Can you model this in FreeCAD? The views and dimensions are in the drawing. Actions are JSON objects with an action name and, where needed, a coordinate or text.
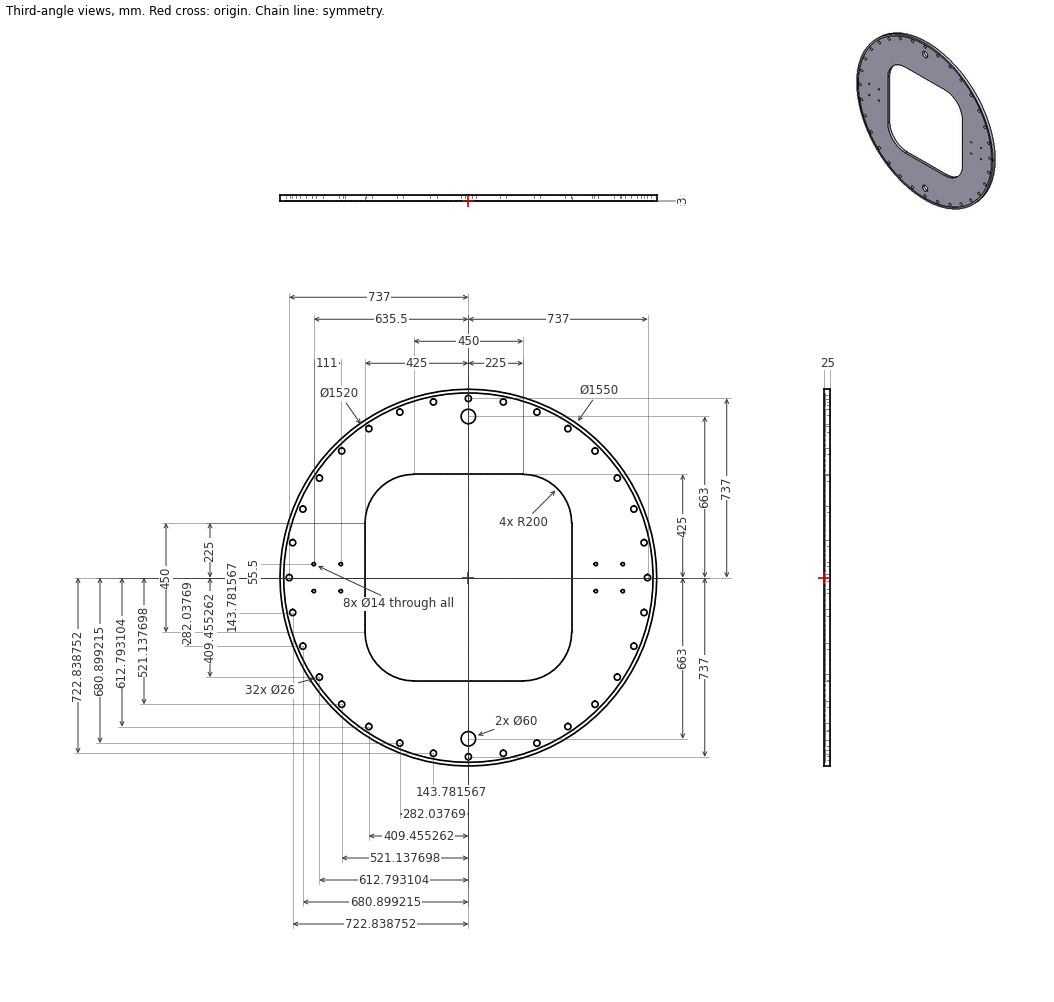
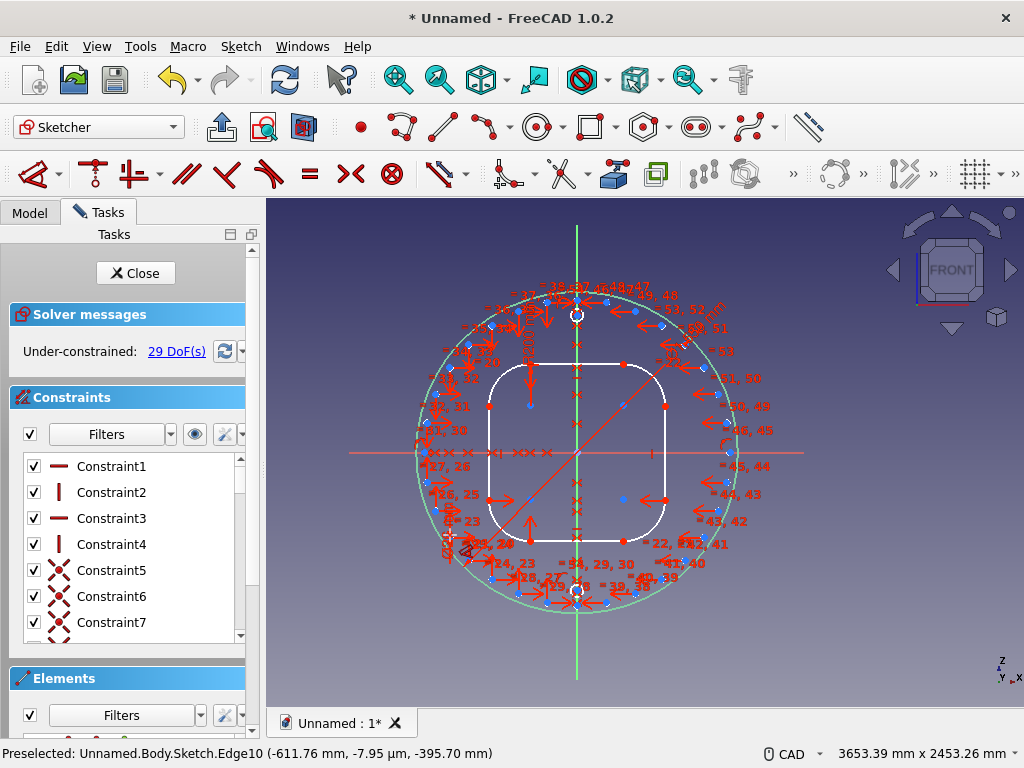
{"action": "scroll", "coordinate": [581, 586], "scroll_direction": "up", "scroll_amount": 6}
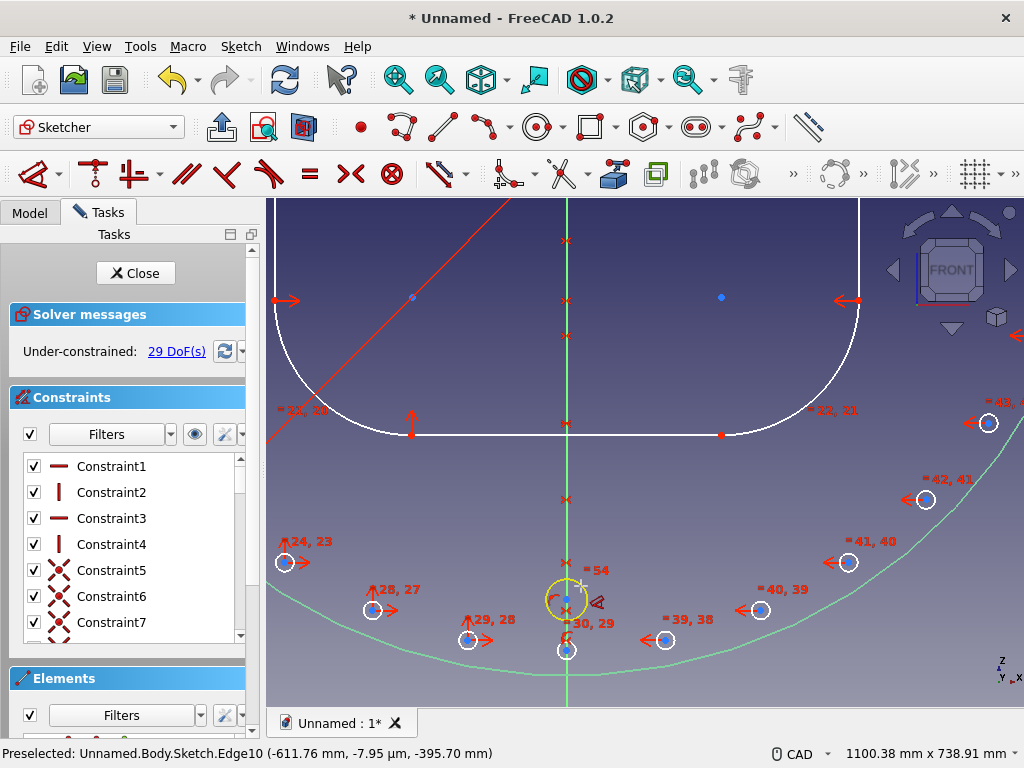
{"action": "left_click", "coordinate": [581, 585]}
{"action": "left_click", "coordinate": [603, 562]}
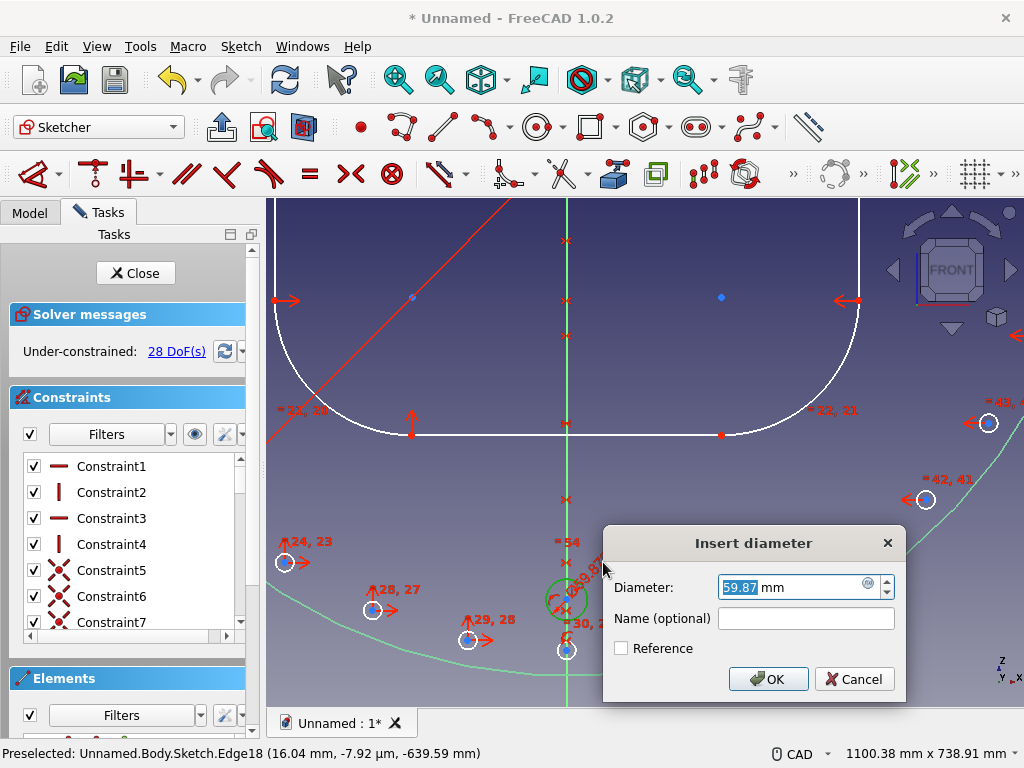
{"action": "type", "text": "60"}
{"action": "key", "text": "Return"}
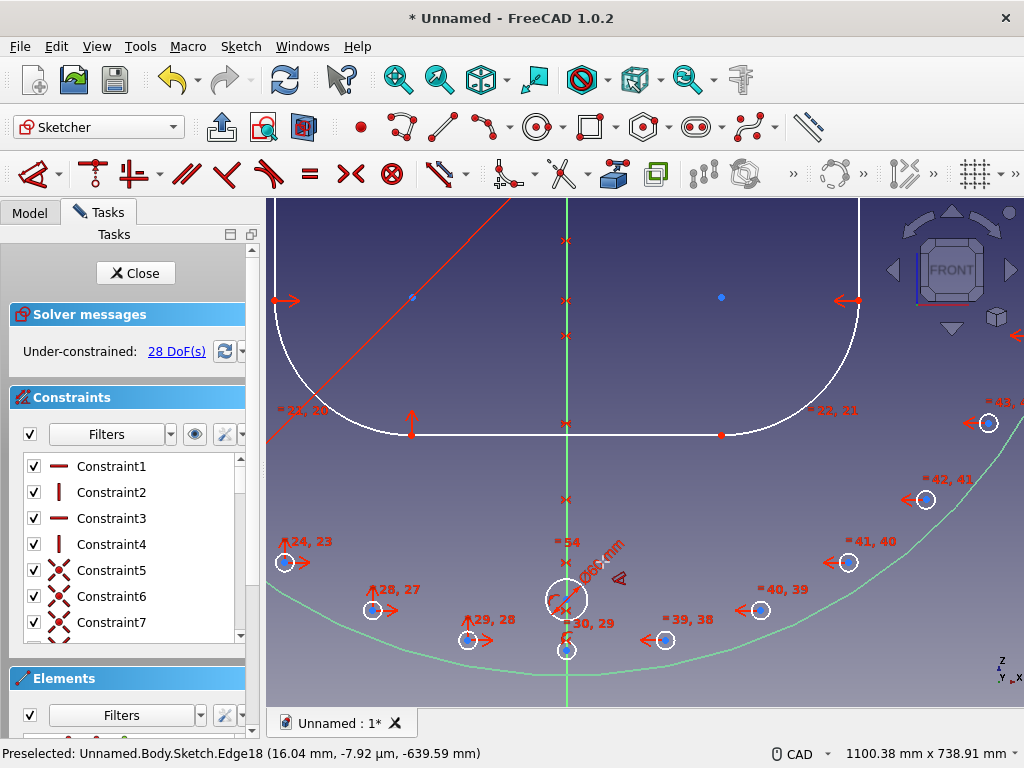
{"action": "scroll", "coordinate": [581, 586], "scroll_direction": "down", "scroll_amount": 6}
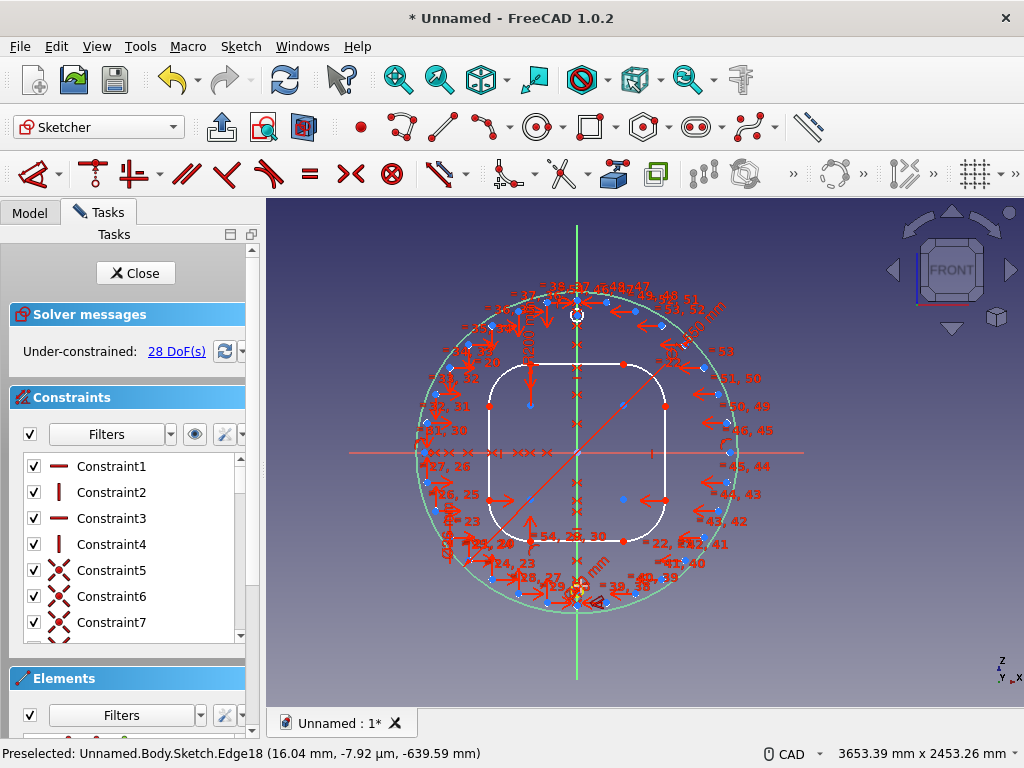
{"action": "left_click", "coordinate": [596, 364]}
{"action": "left_click", "coordinate": [610, 330]}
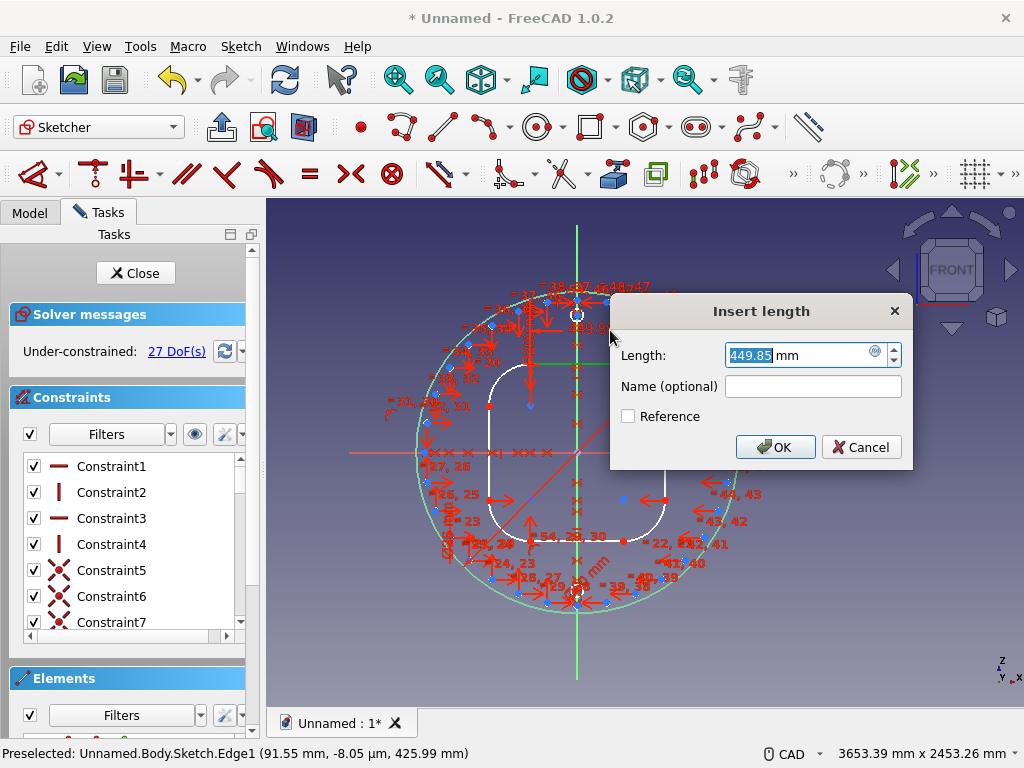
{"action": "type", "text": "450"}
{"action": "key", "text": "Return"}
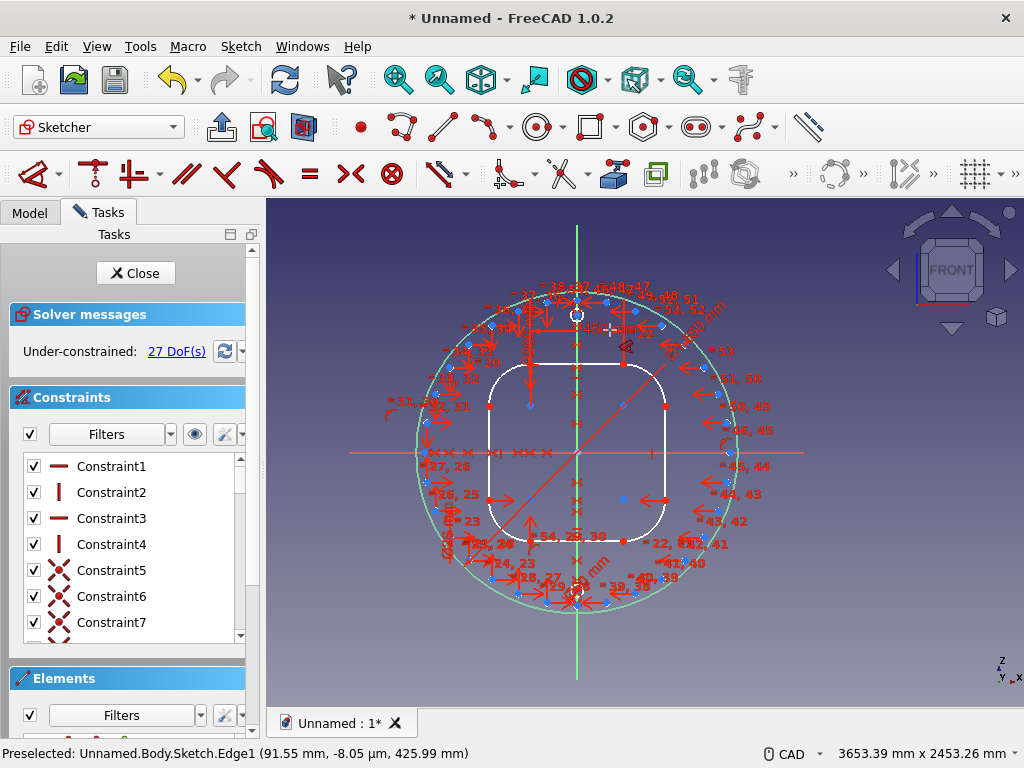
{"action": "left_click", "coordinate": [489, 435]}
{"action": "left_click", "coordinate": [455, 432]}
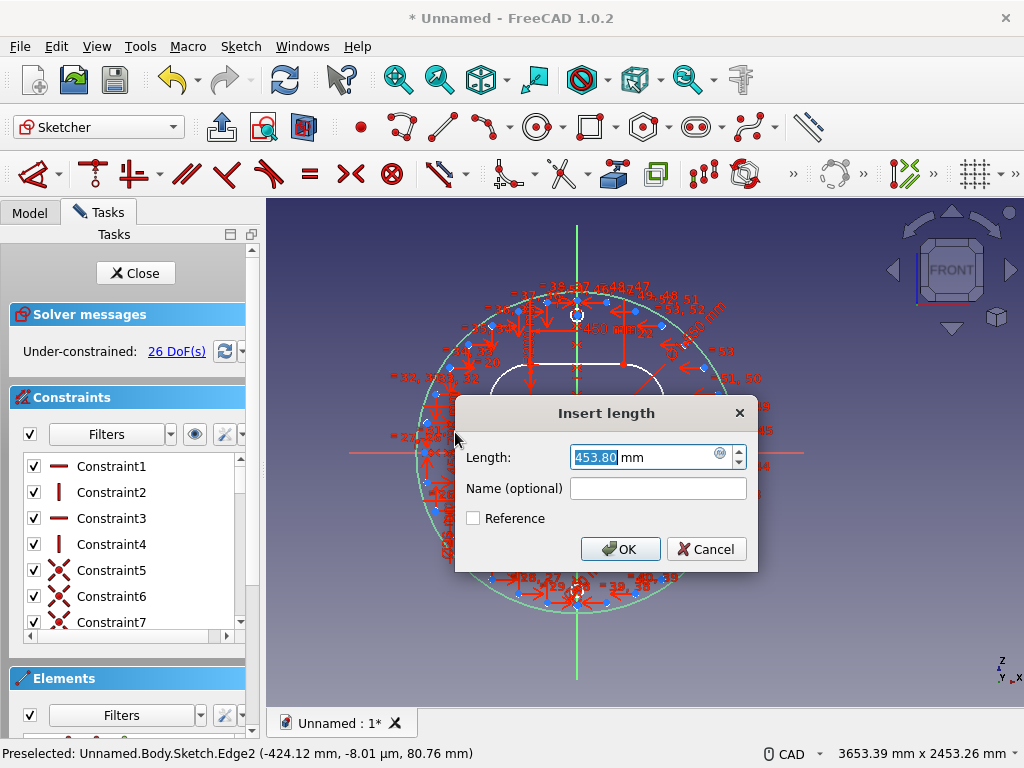
{"action": "type", "text": "450"}
{"action": "key", "text": "Return"}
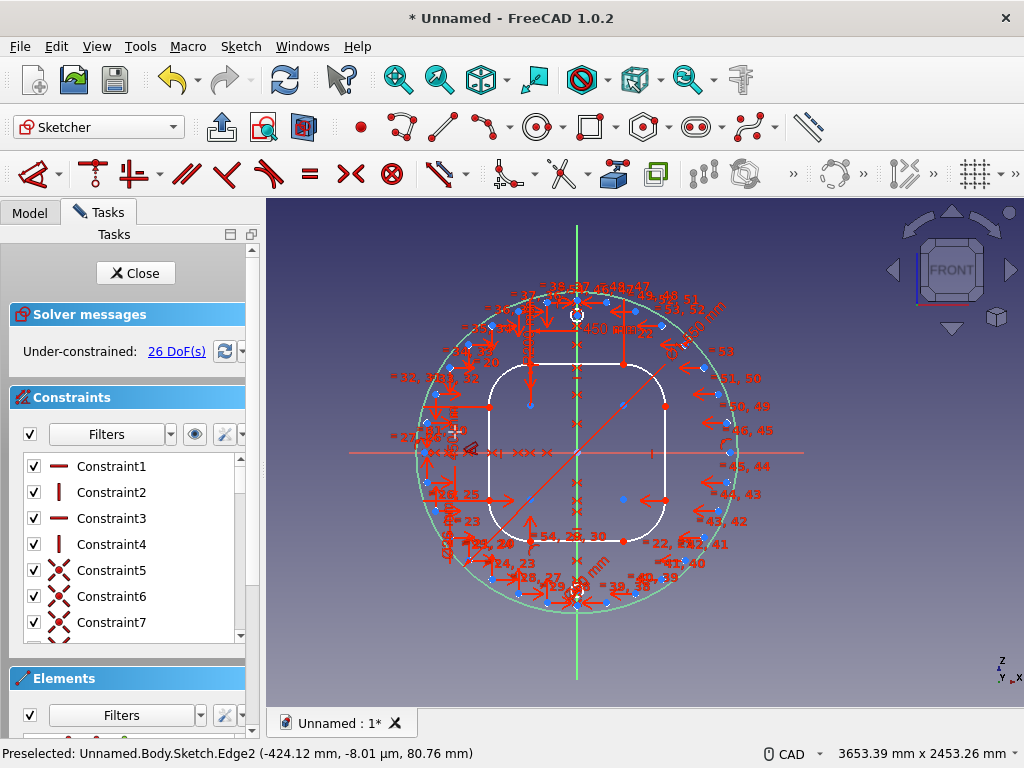
{"action": "left_click", "coordinate": [558, 541]}
{"action": "left_click", "coordinate": [556, 507]}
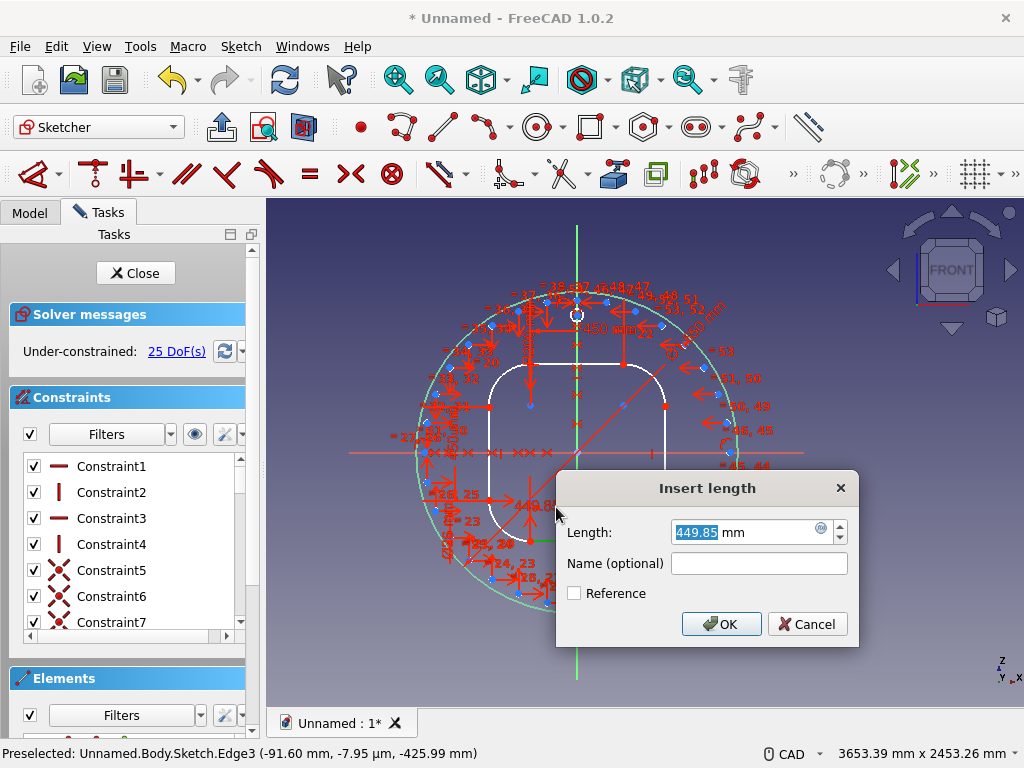
{"action": "type", "text": "450"}
{"action": "key", "text": "Return"}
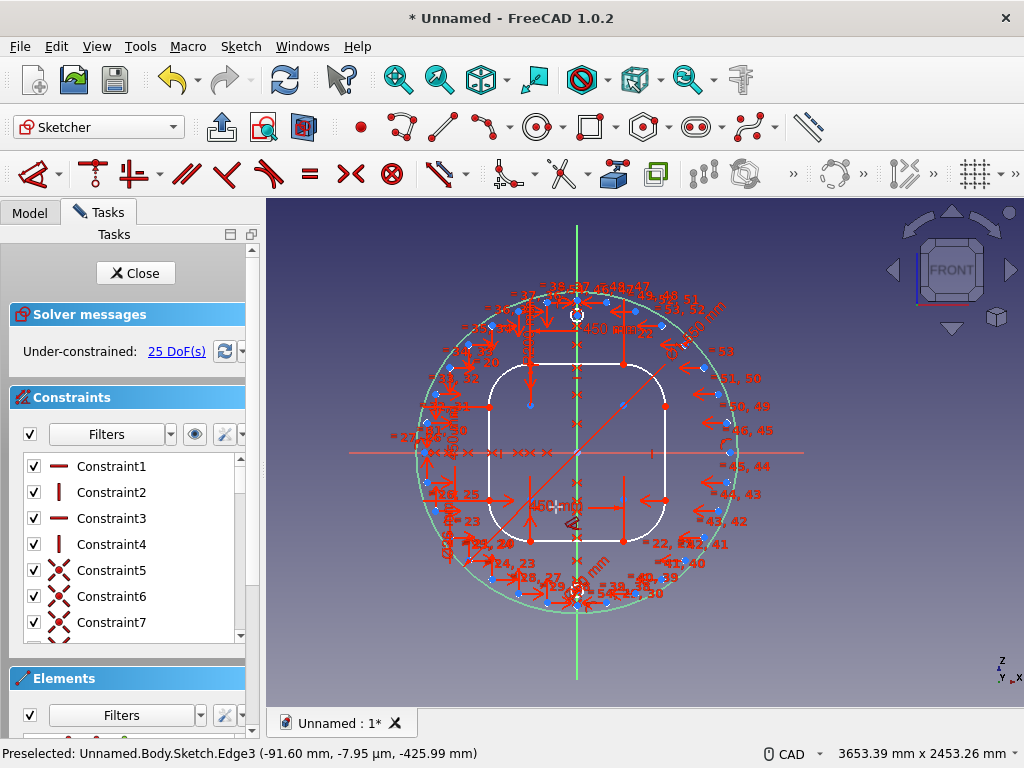
{"action": "left_click", "coordinate": [665, 472]}
{"action": "left_click", "coordinate": [699, 432]}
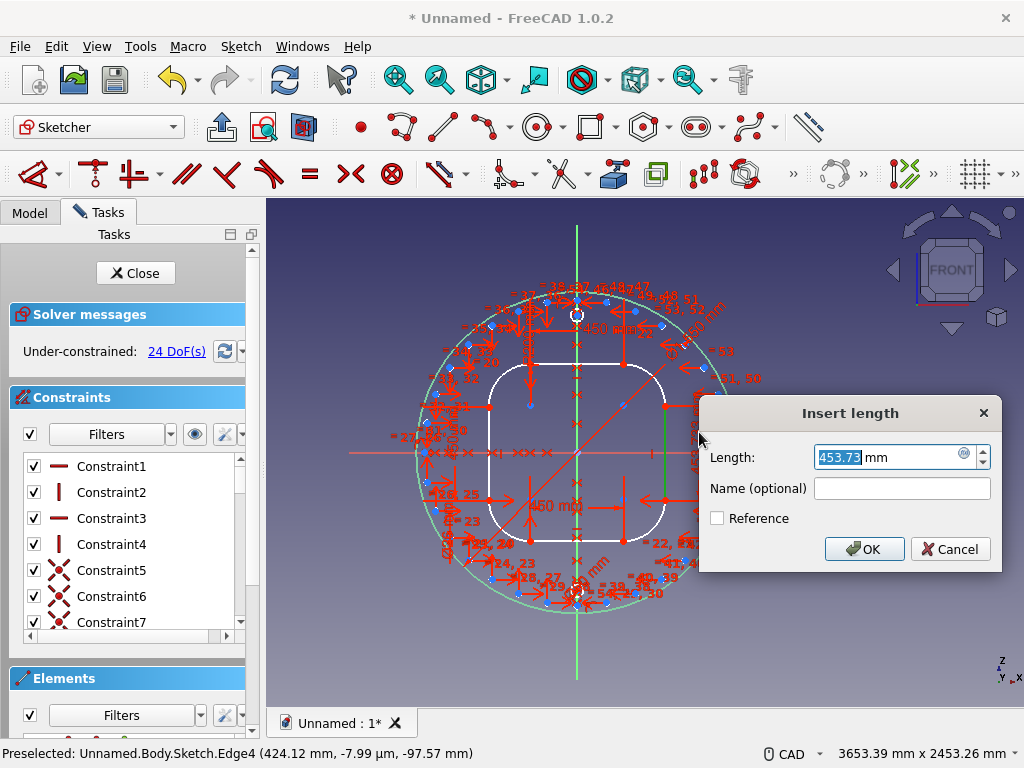
{"action": "type", "text": "450"}
{"action": "key", "text": "Return"}